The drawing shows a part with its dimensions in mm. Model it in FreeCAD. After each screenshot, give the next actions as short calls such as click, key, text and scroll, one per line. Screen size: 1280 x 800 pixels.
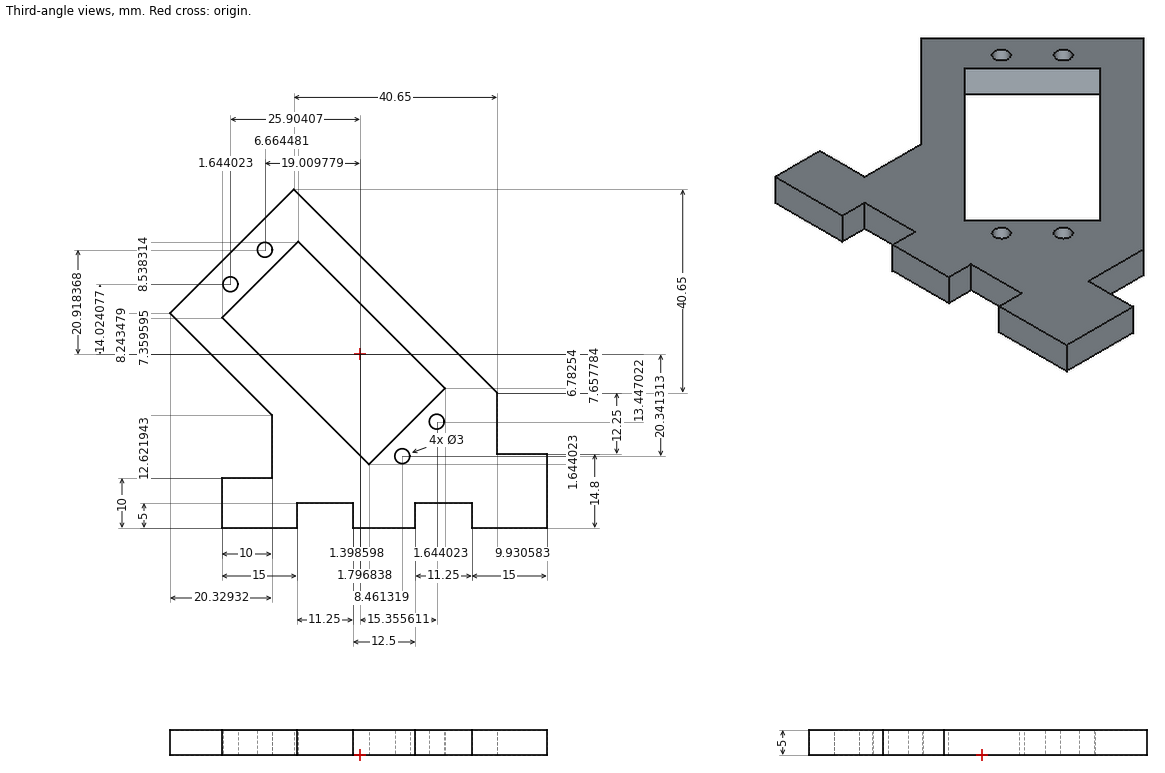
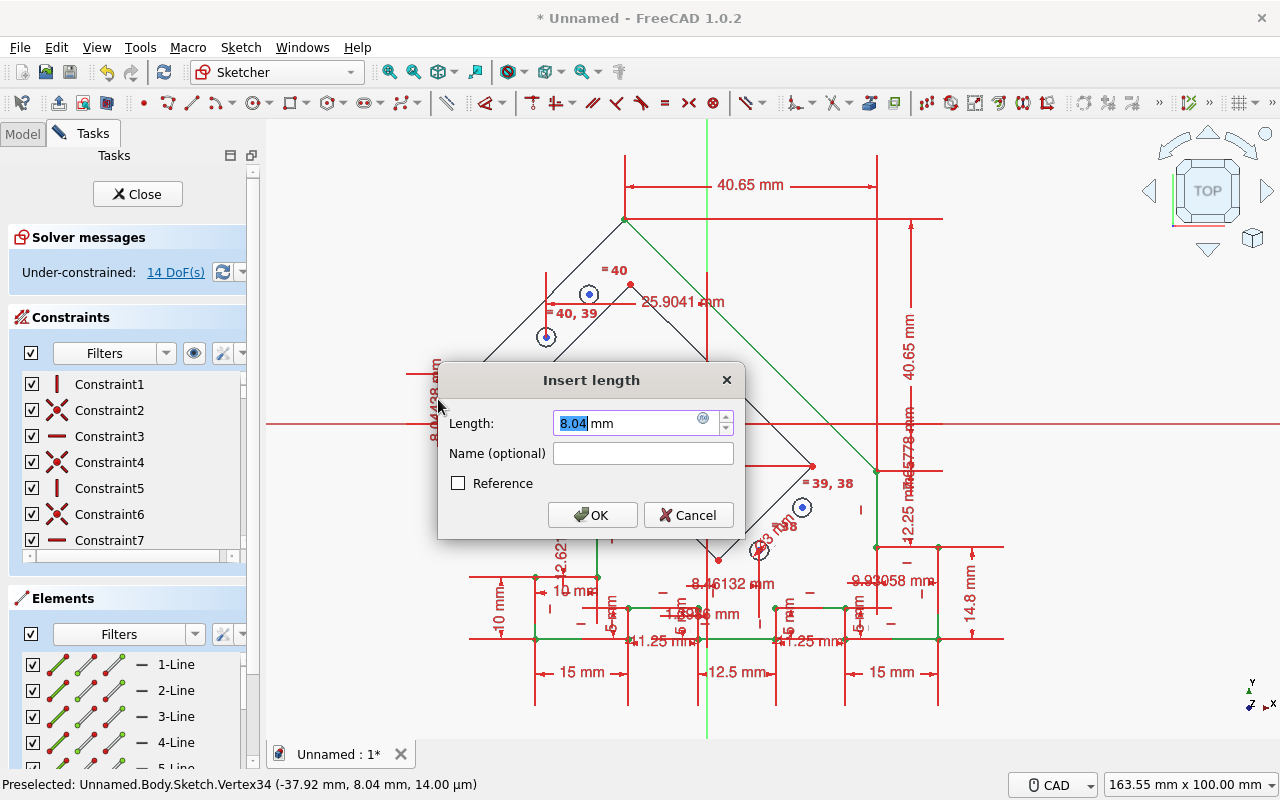
text(8.243479)
key(Return)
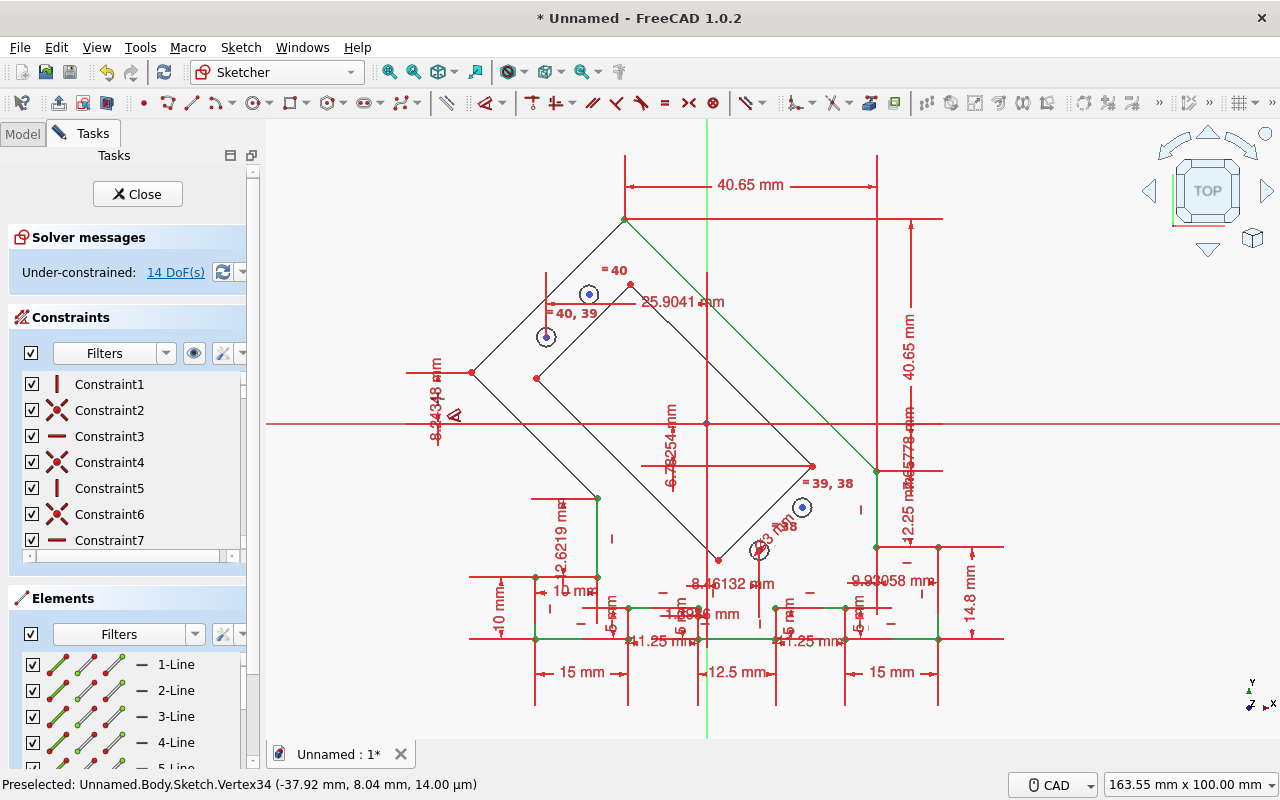
scroll(718, 561, up, 7)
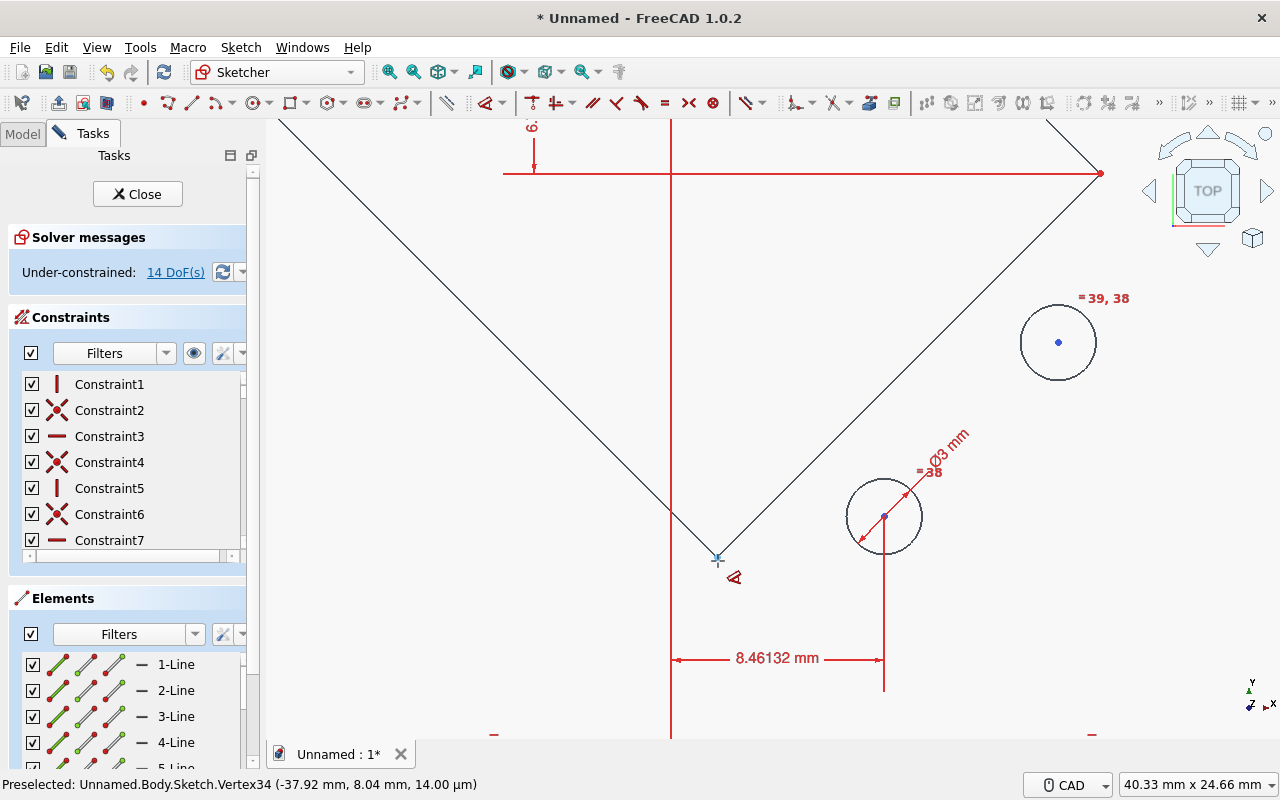
click(717, 558)
click(694, 592)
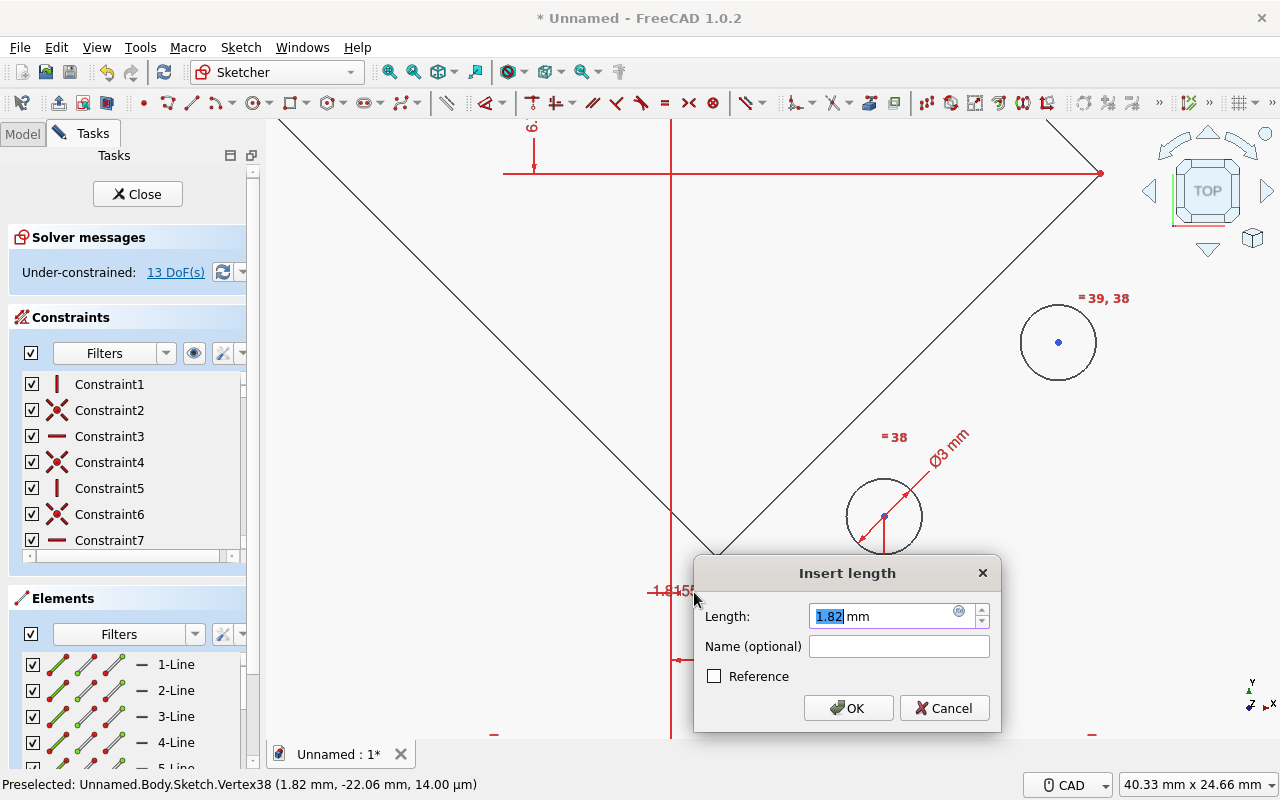
text(1.796838)
key(Return)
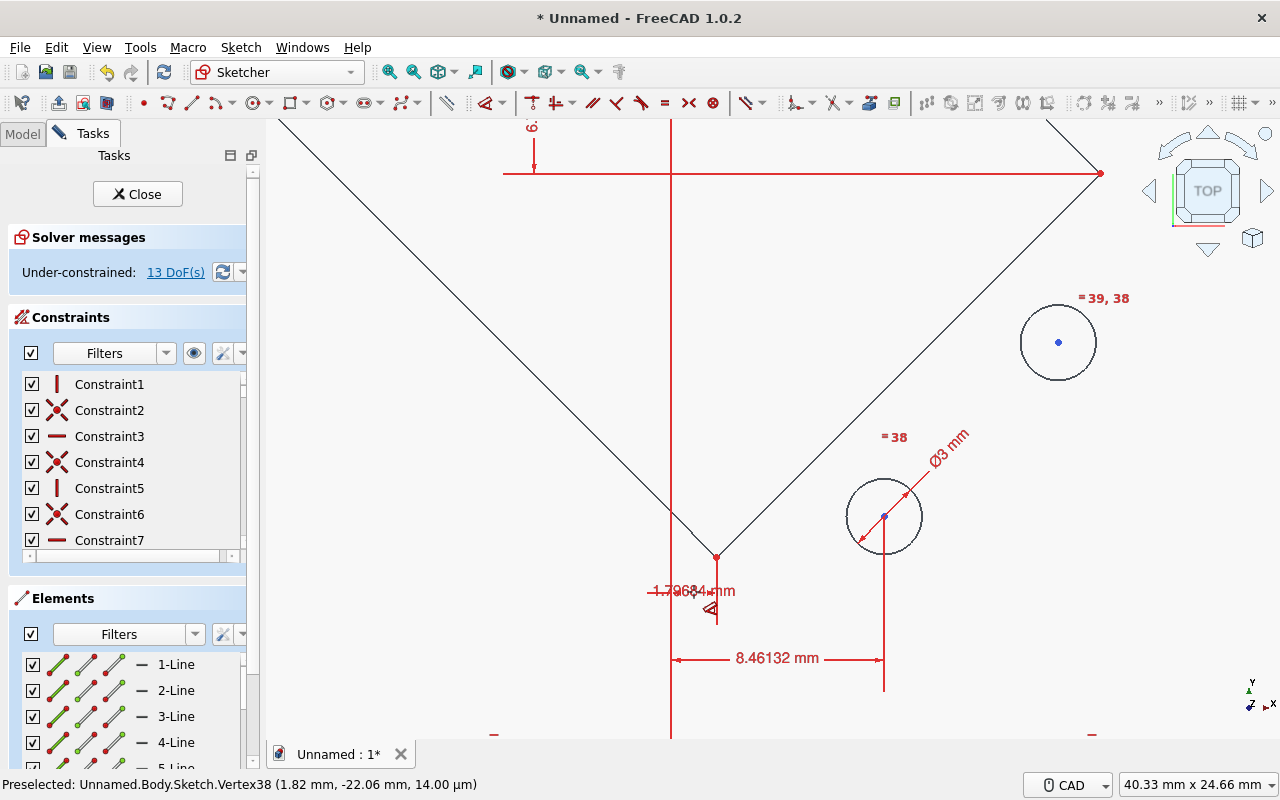
scroll(718, 561, down, 7)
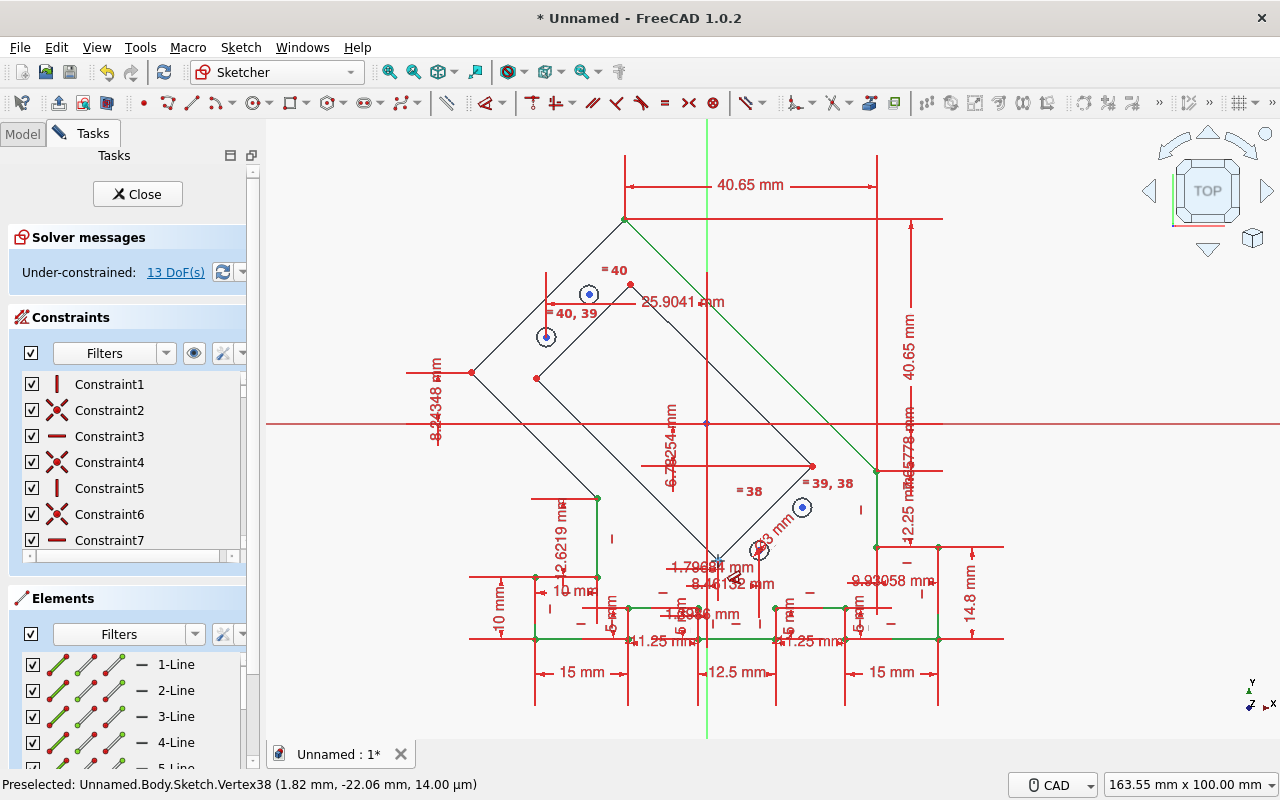
click(536, 379)
click(765, 391)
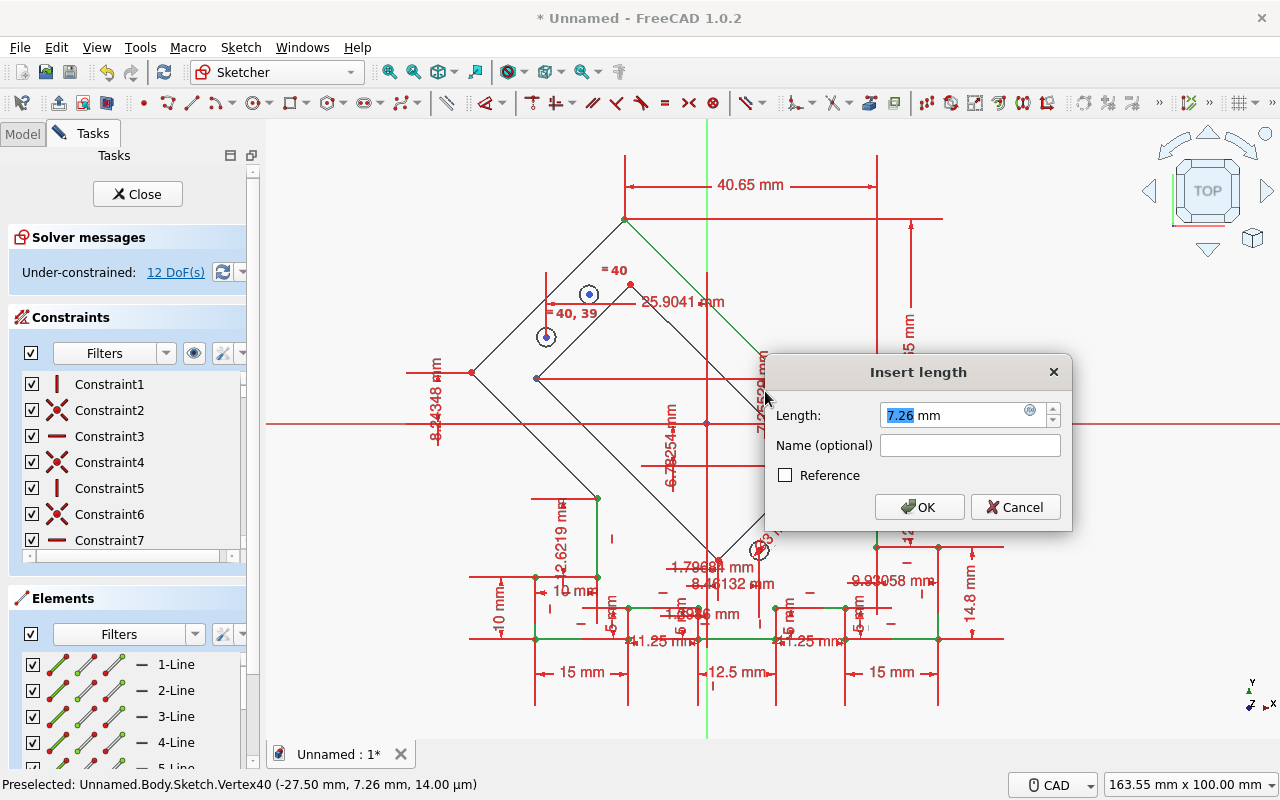
text(7.359595)
key(Return)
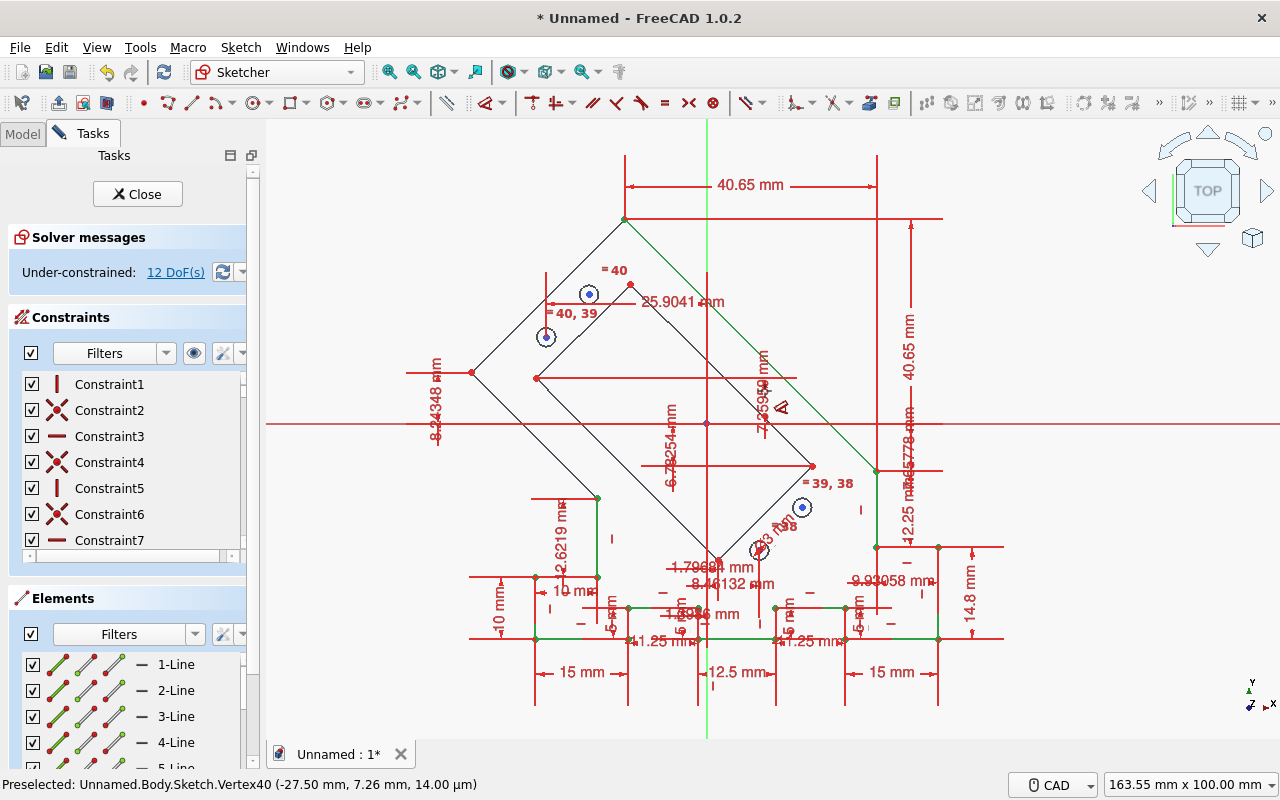
click(509, 411)
click(491, 533)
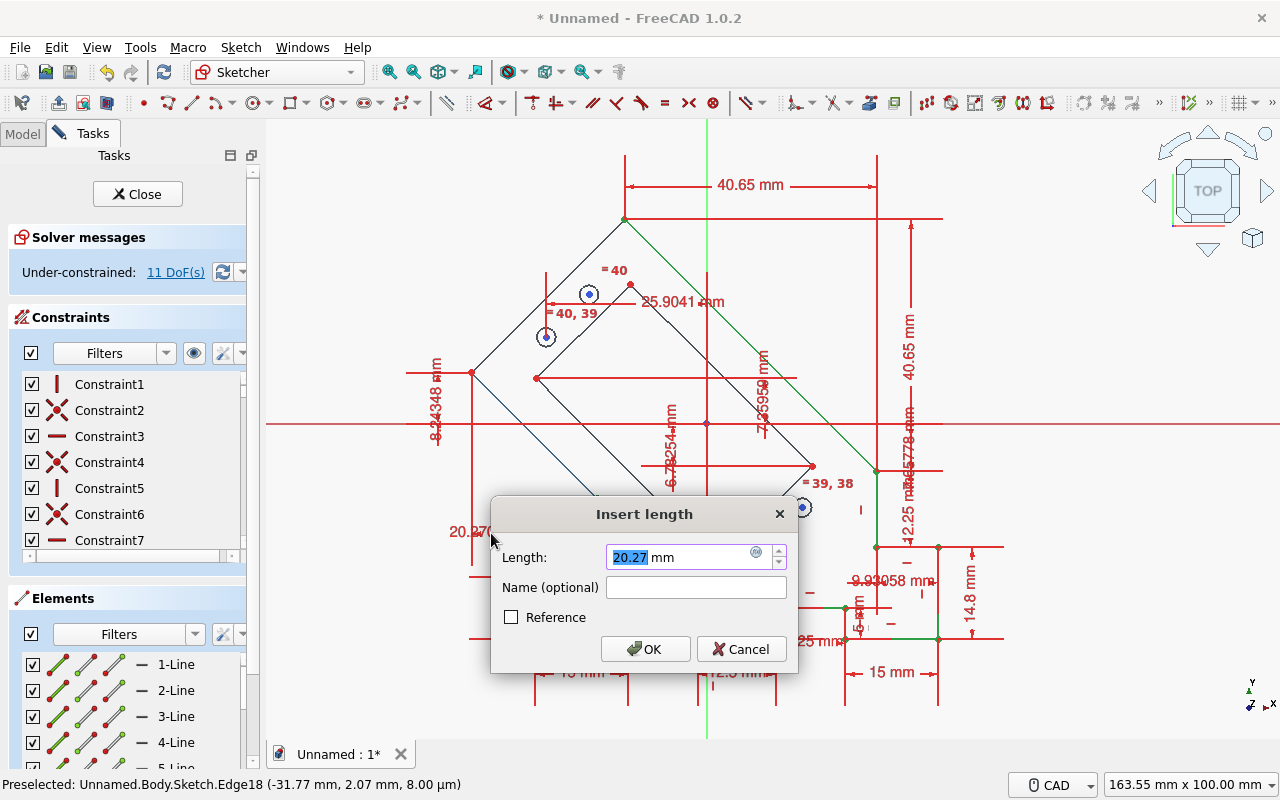
text(20.32932)
key(Return)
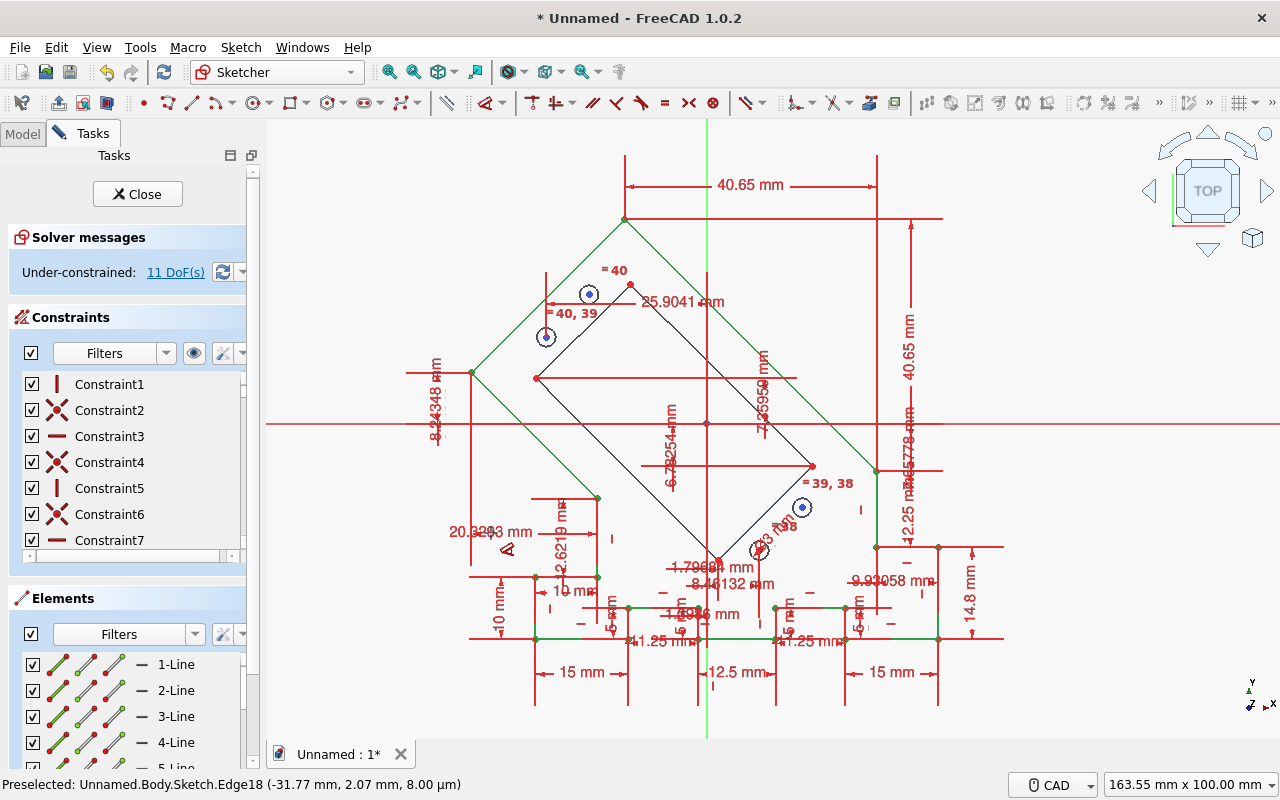
click(759, 551)
click(673, 487)